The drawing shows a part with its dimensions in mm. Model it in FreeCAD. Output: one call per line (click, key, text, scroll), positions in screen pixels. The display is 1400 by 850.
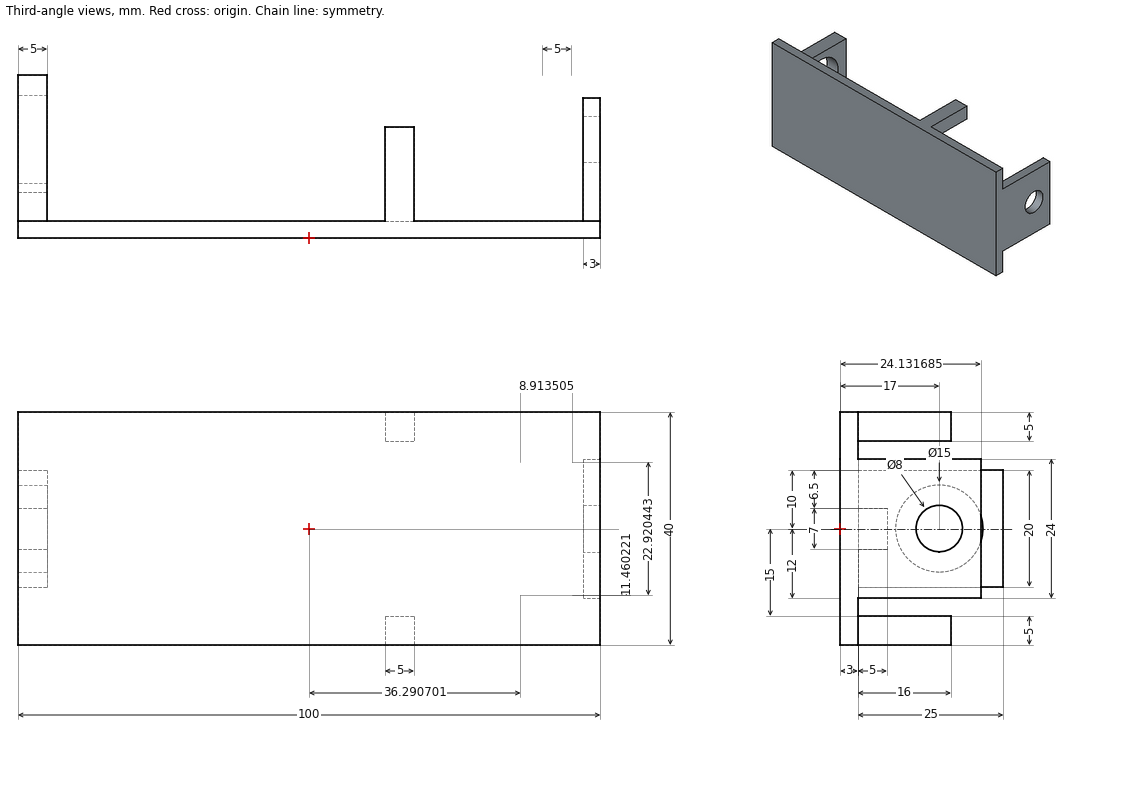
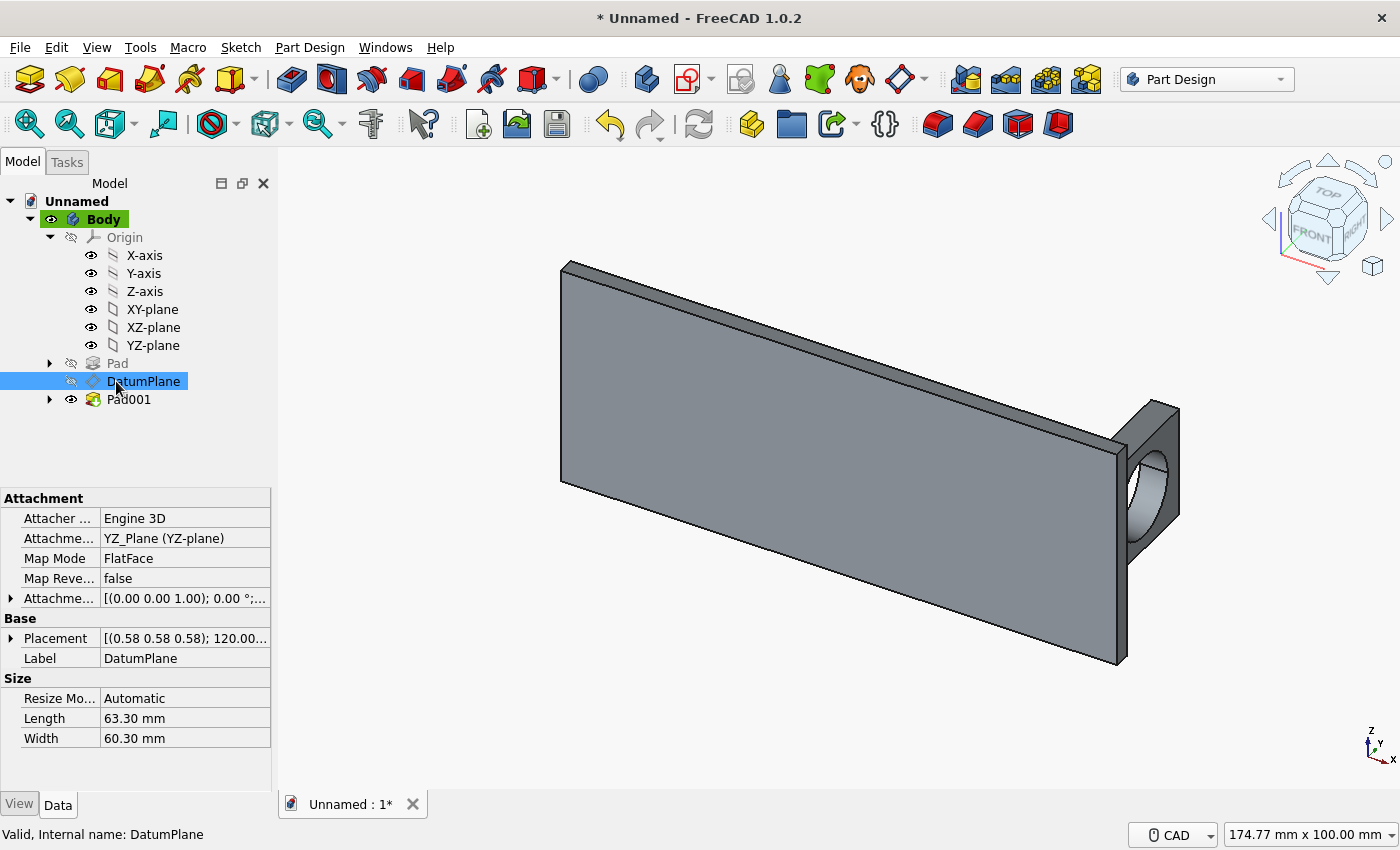
key(6)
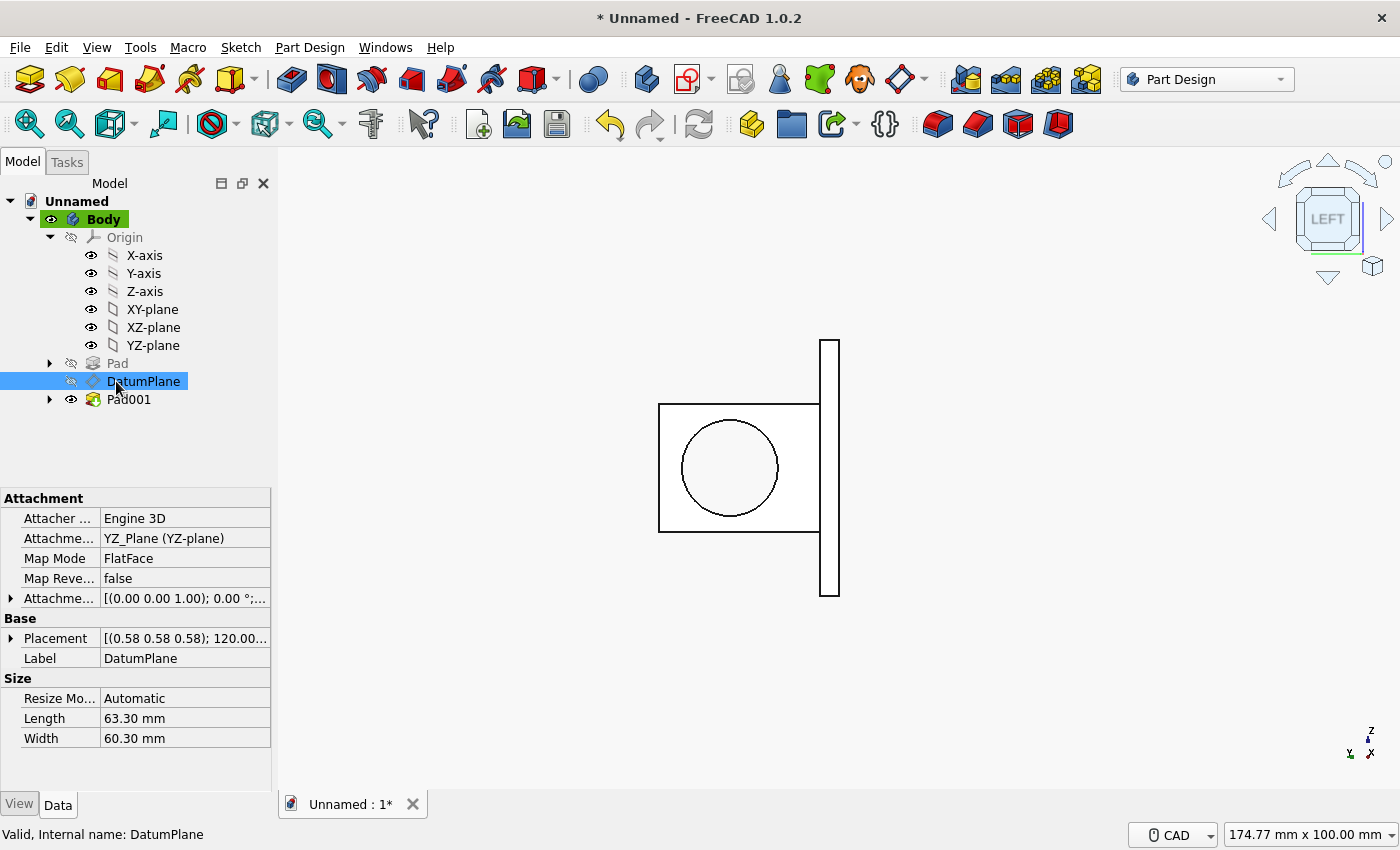
click(30, 124)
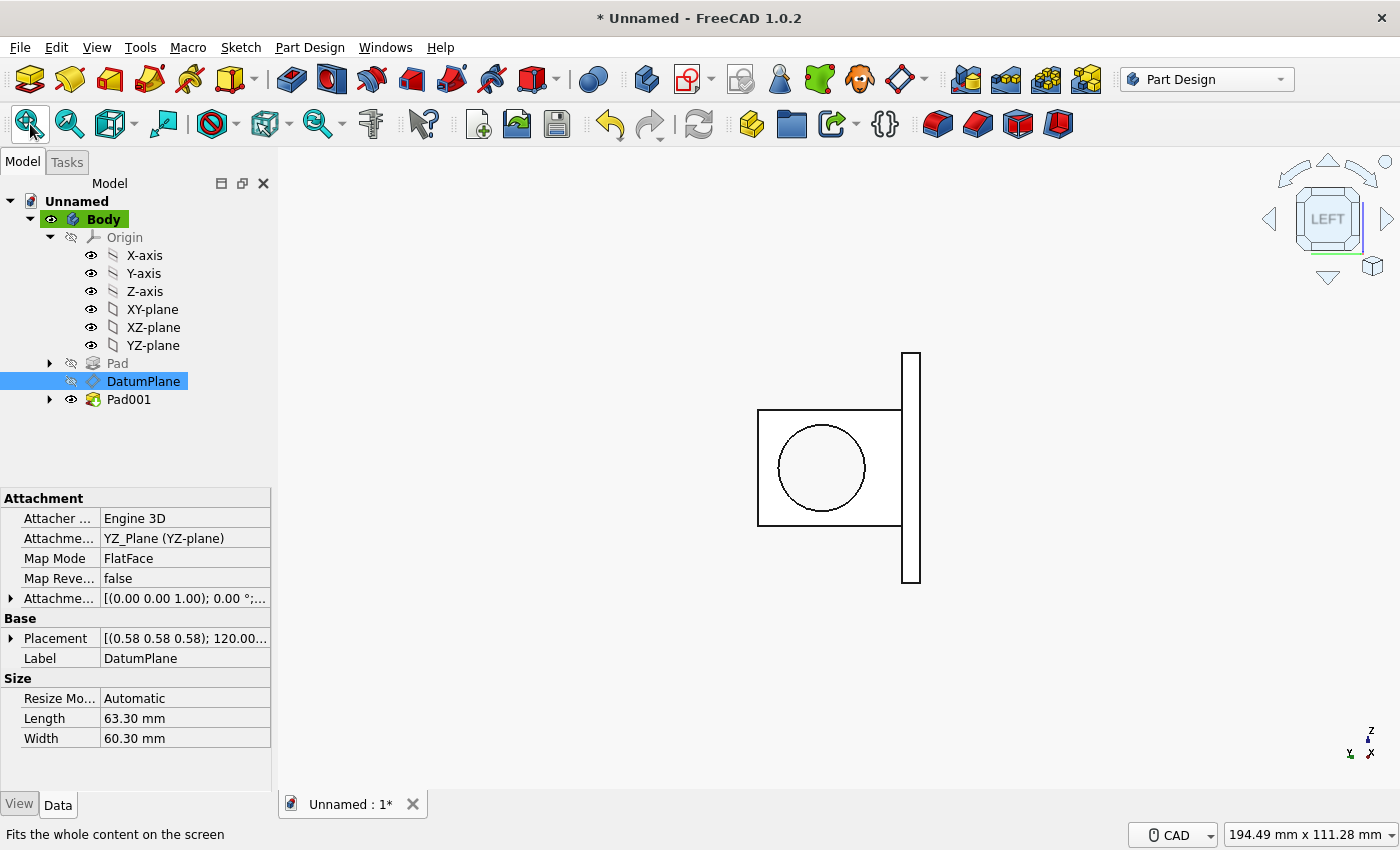
click(911, 368)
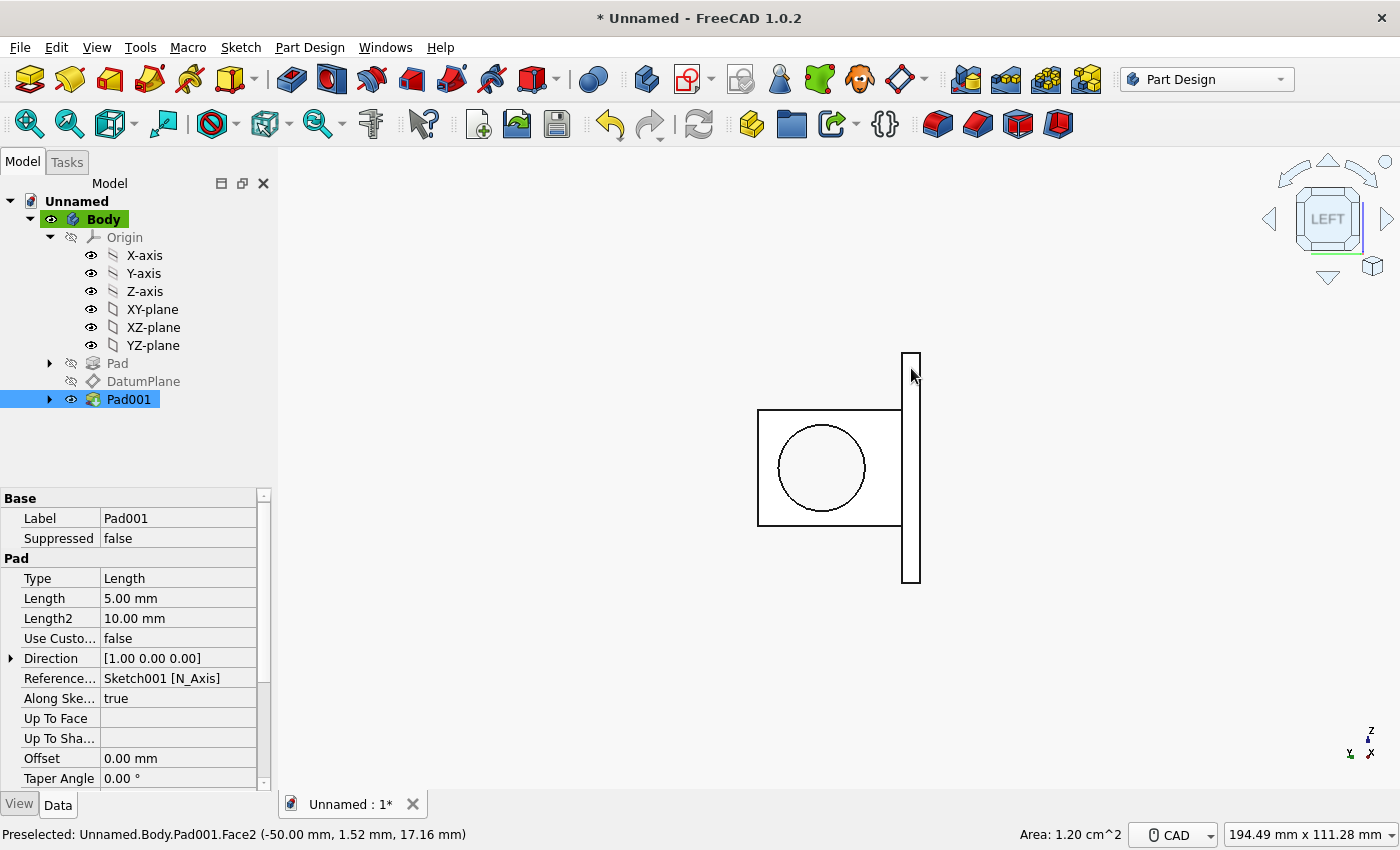
click(688, 80)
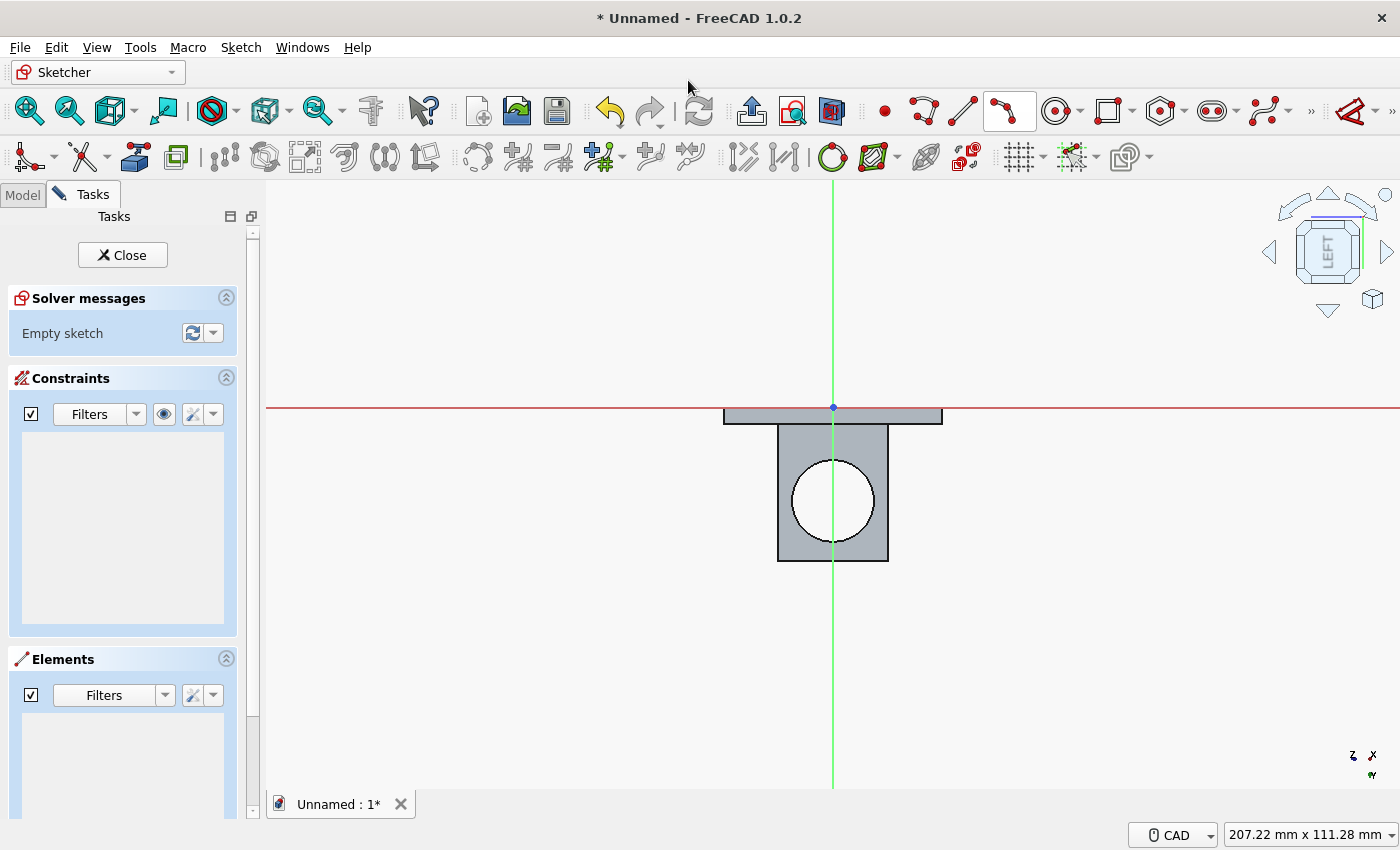
scroll(873, 484, up, 5)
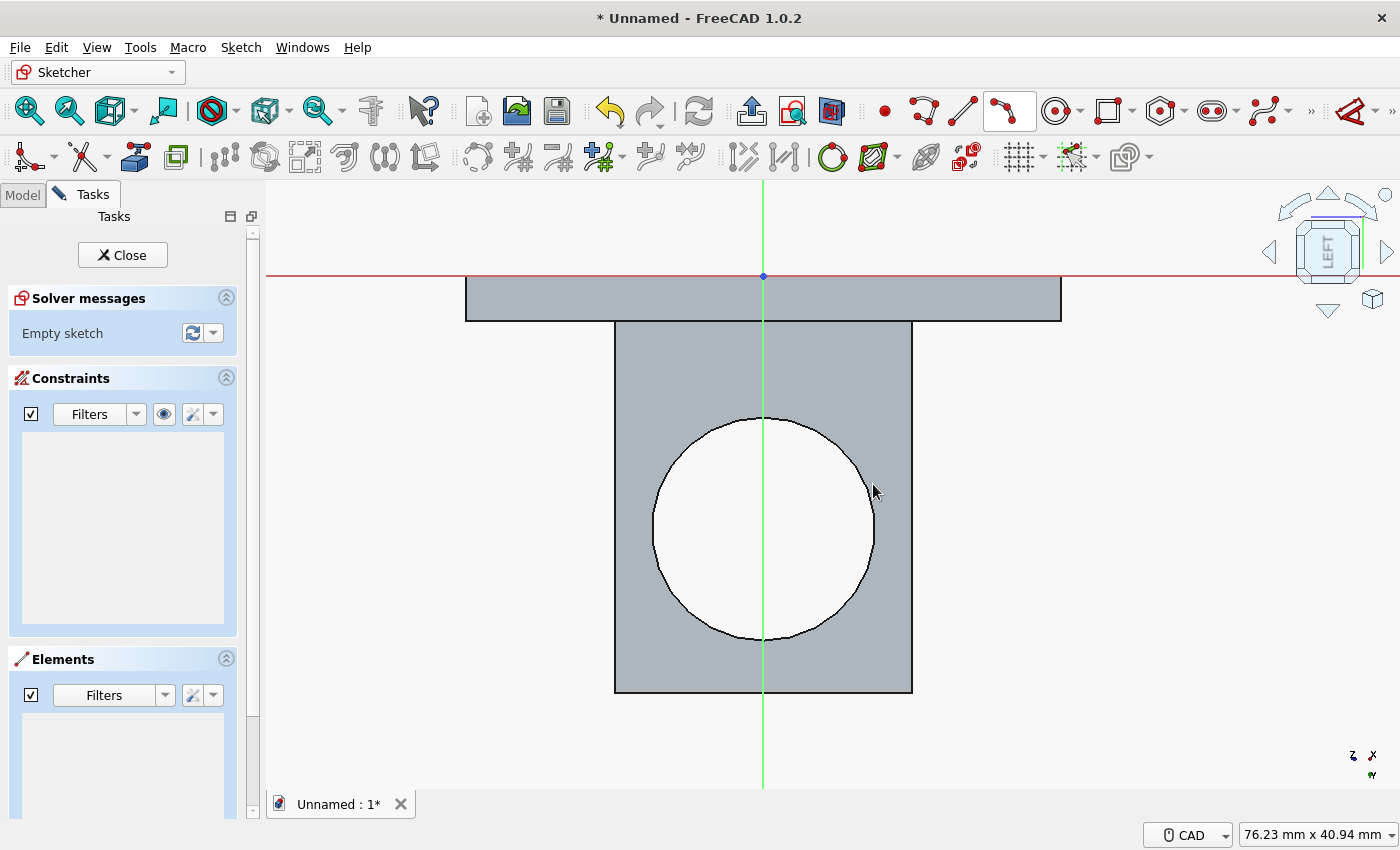
click(924, 112)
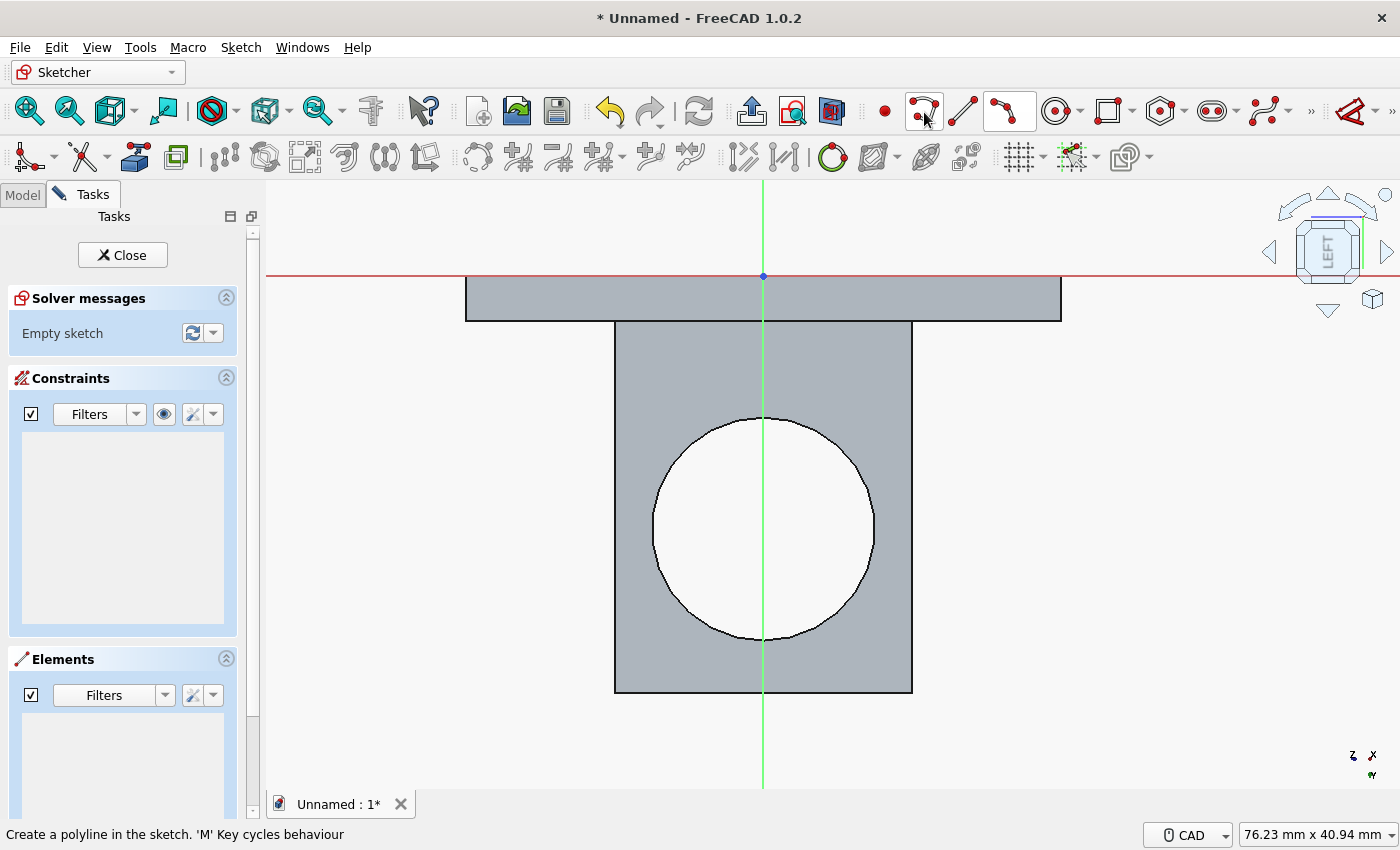
click(815, 321)
click(815, 395)
click(711, 395)
click(711, 321)
click(615, 321)
click(615, 693)
click(912, 693)
click(912, 321)
click(815, 322)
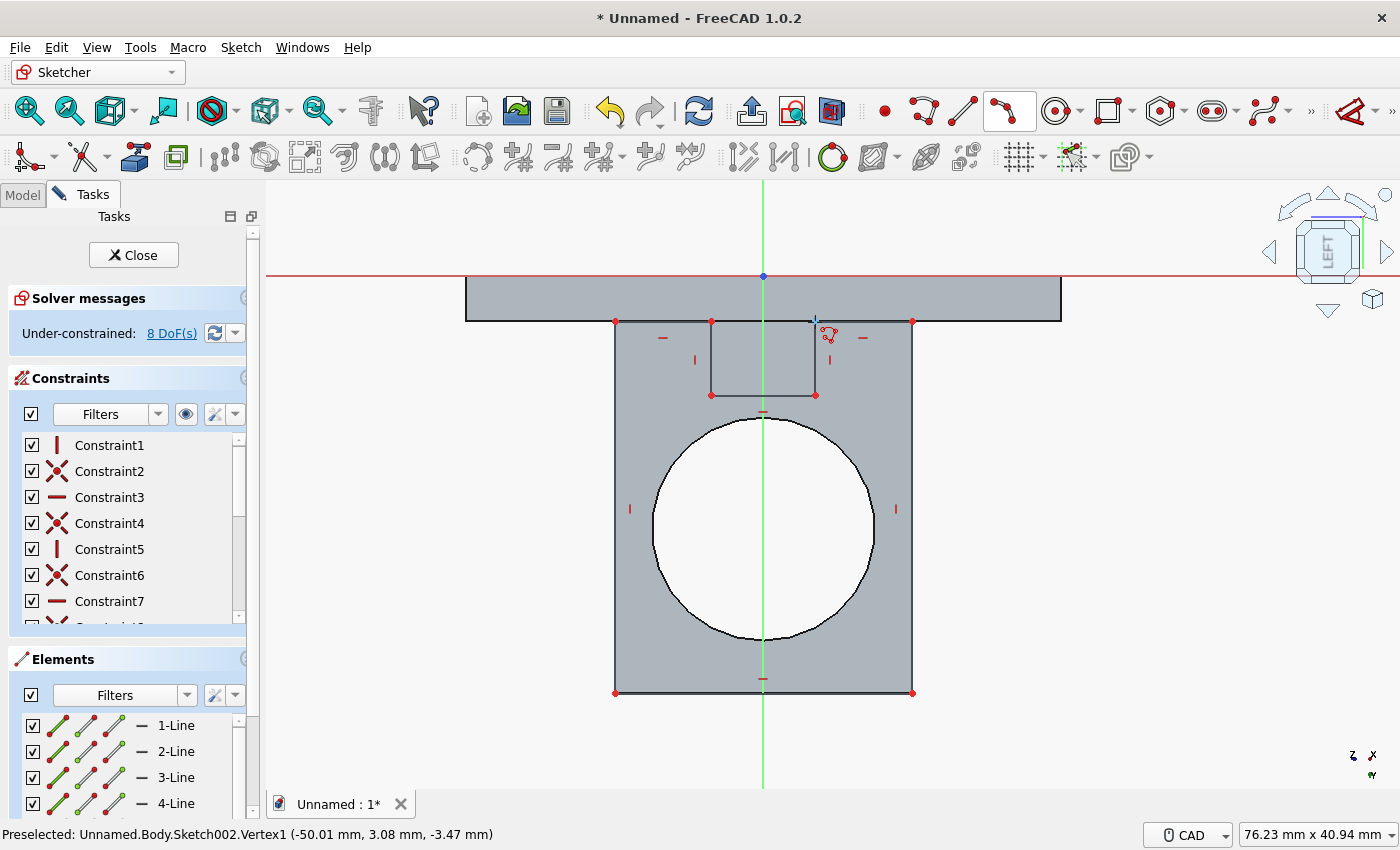
click(1056, 112)